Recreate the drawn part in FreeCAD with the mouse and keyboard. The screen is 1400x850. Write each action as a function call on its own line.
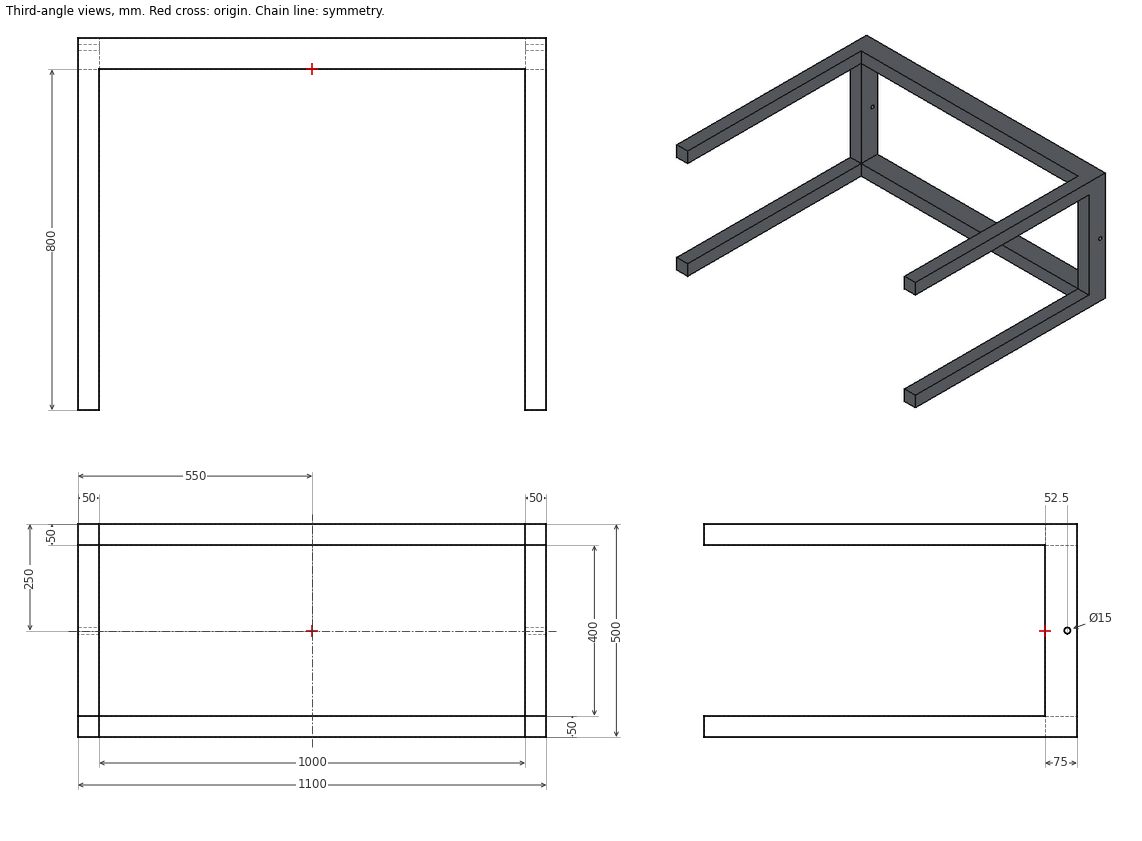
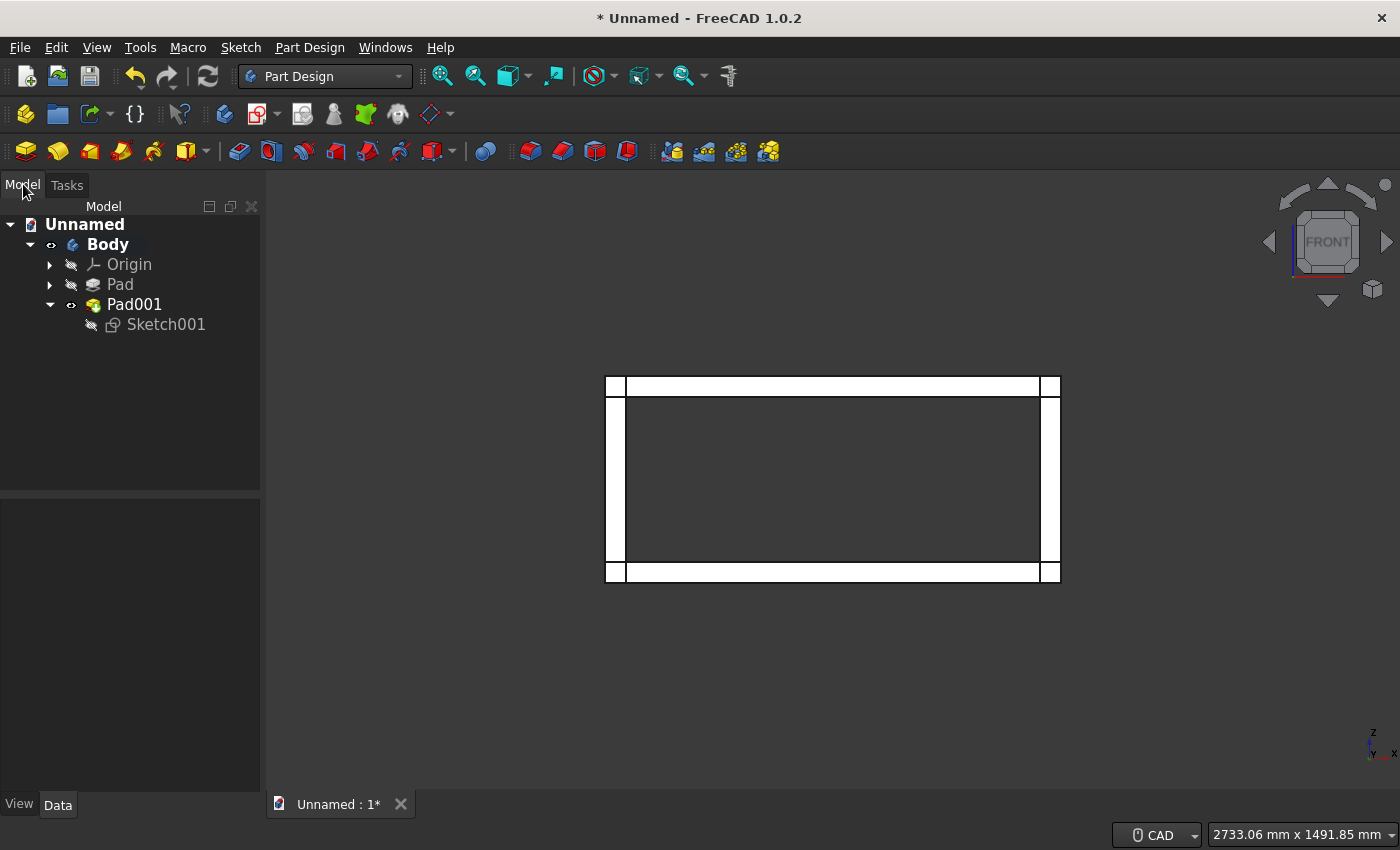
click(50, 265)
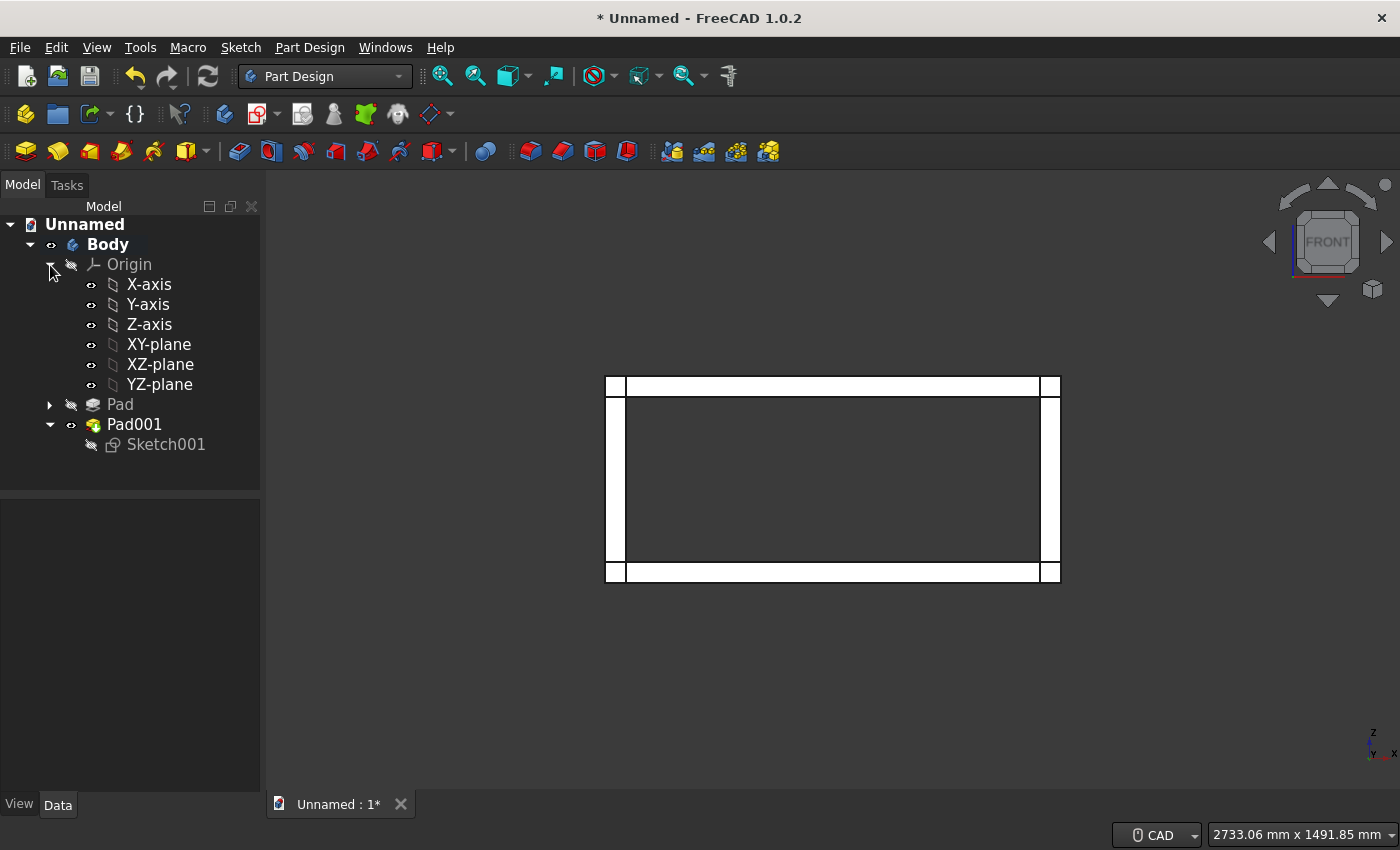
click(136, 385)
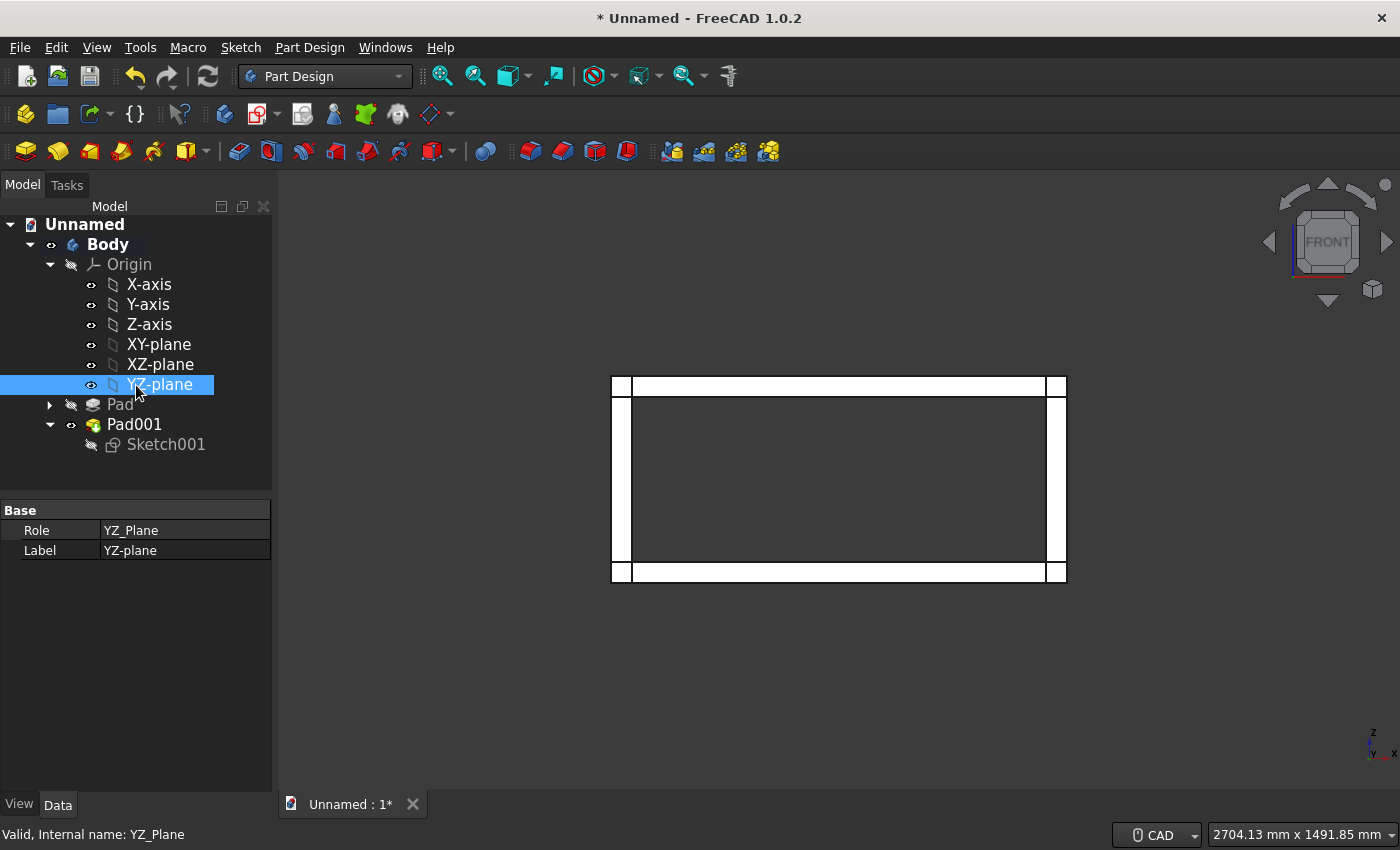
click(430, 114)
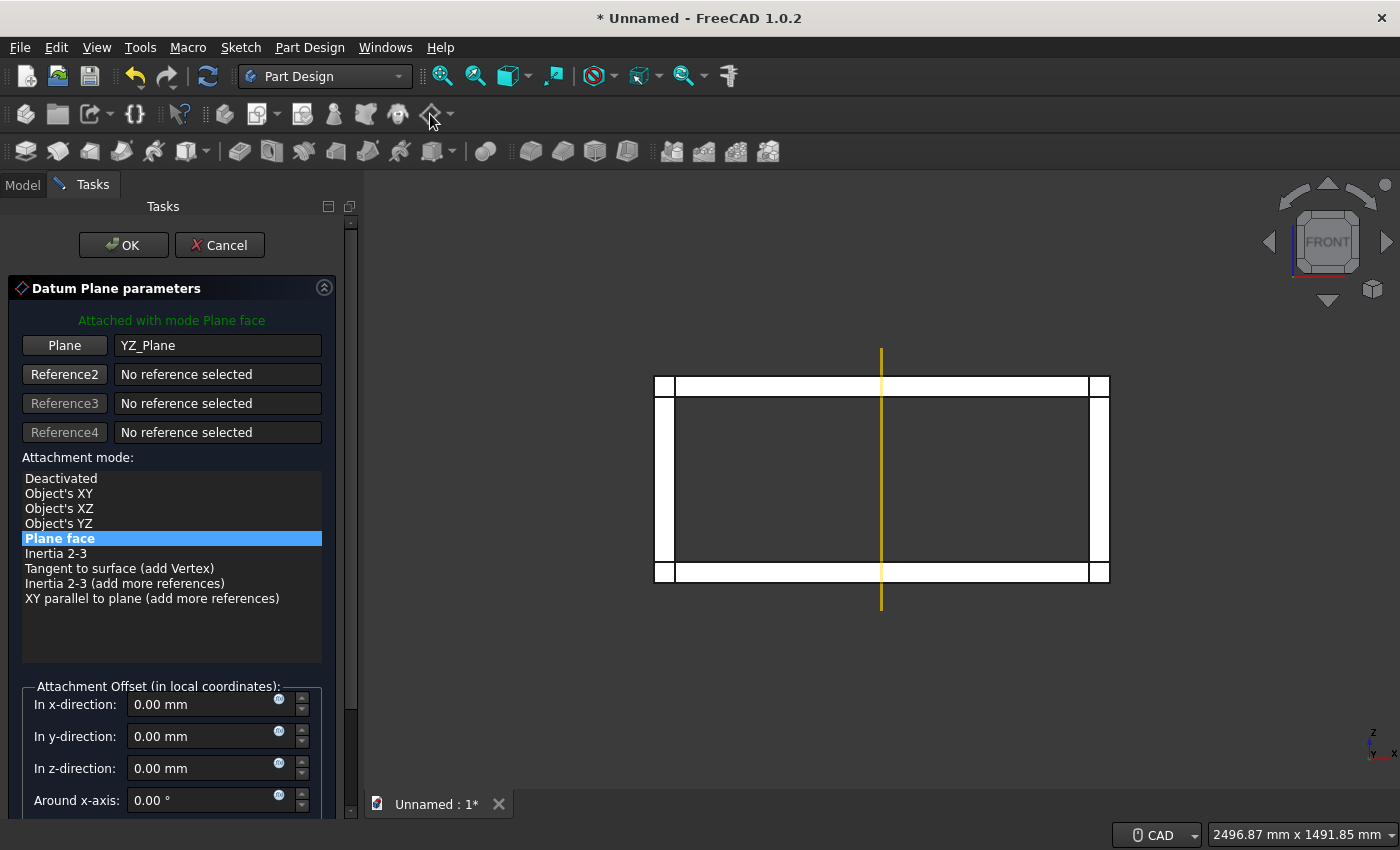
triple_click(210, 768)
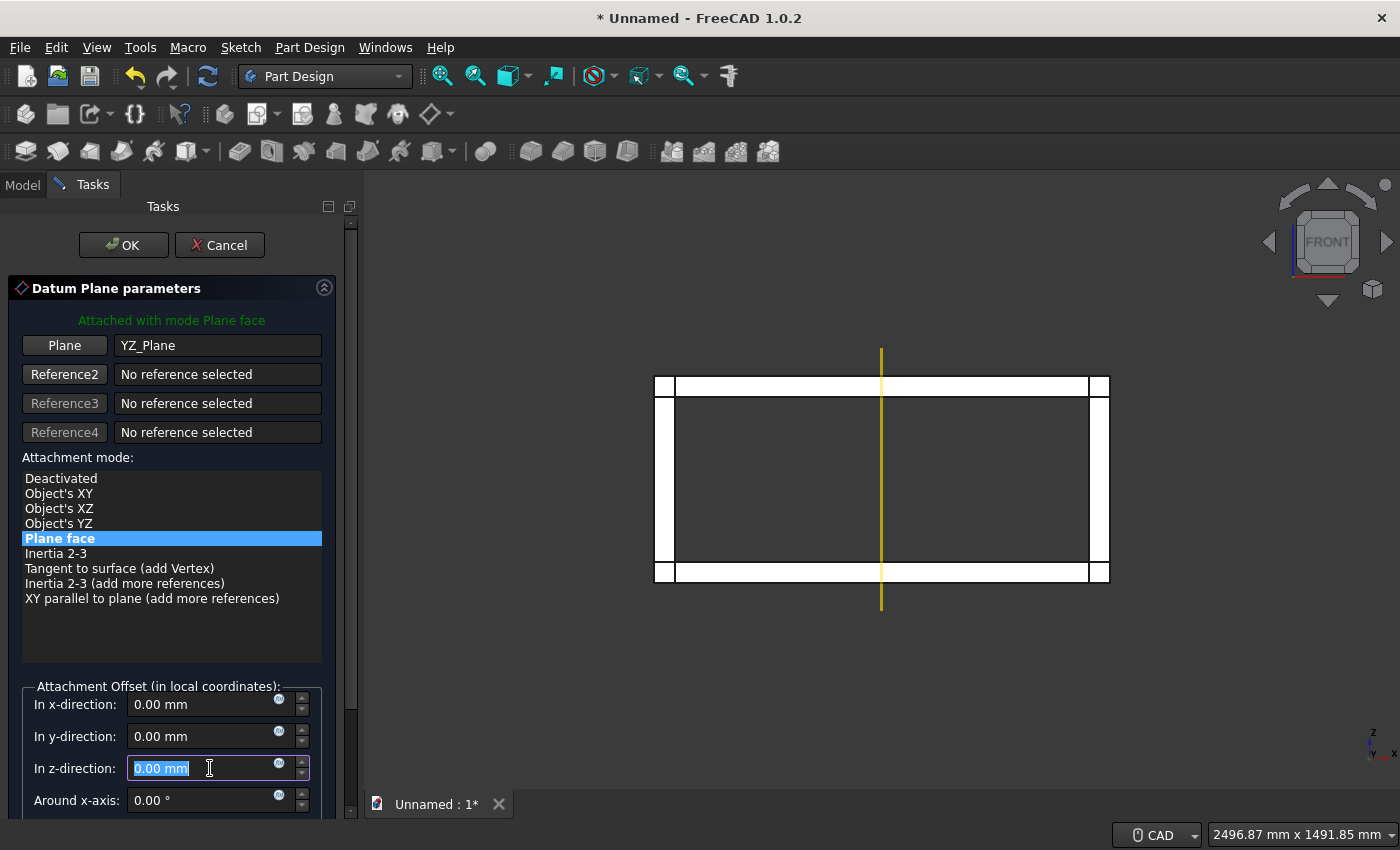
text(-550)
key(Tab)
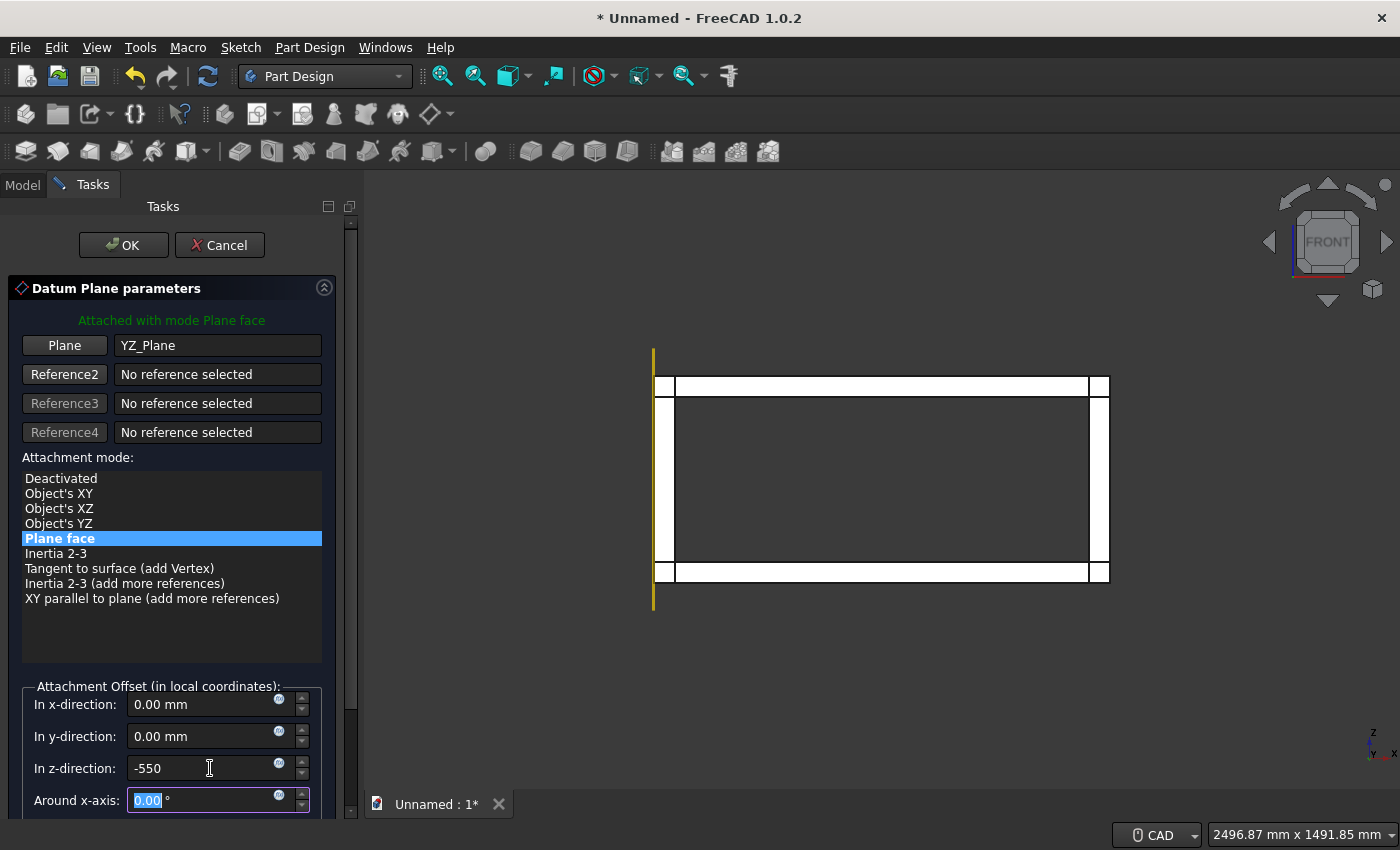
click(124, 245)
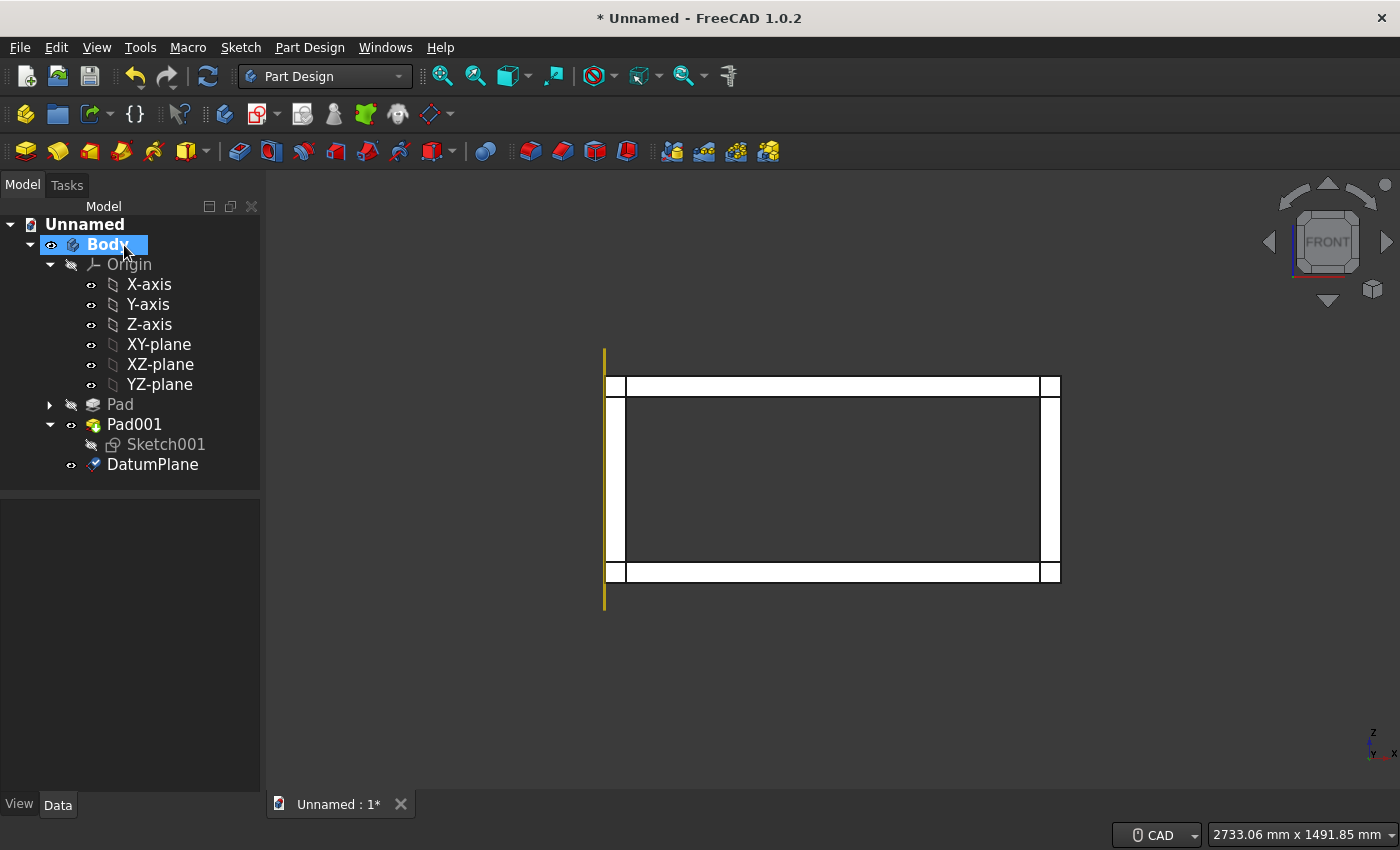
click(116, 465)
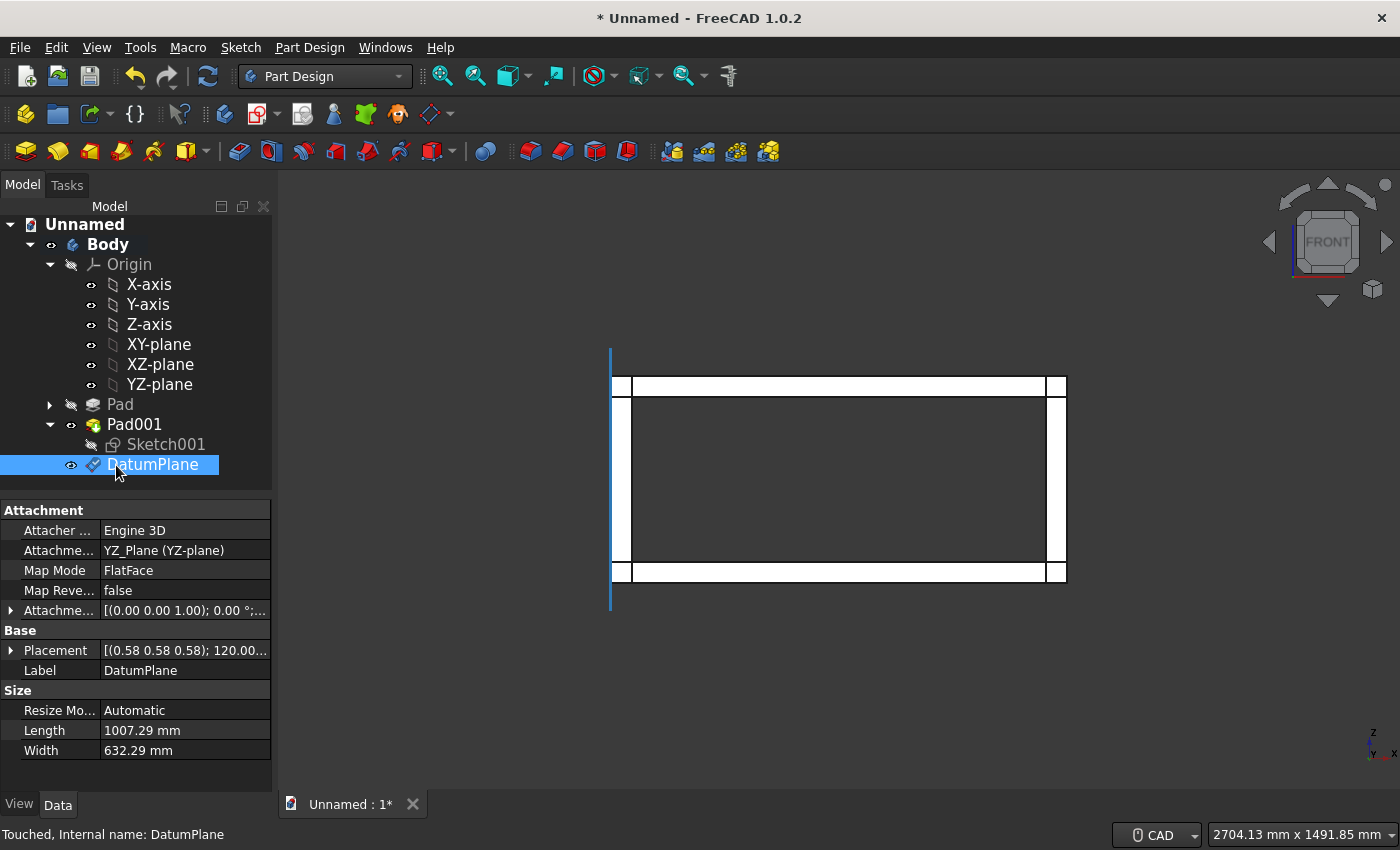
click(258, 114)